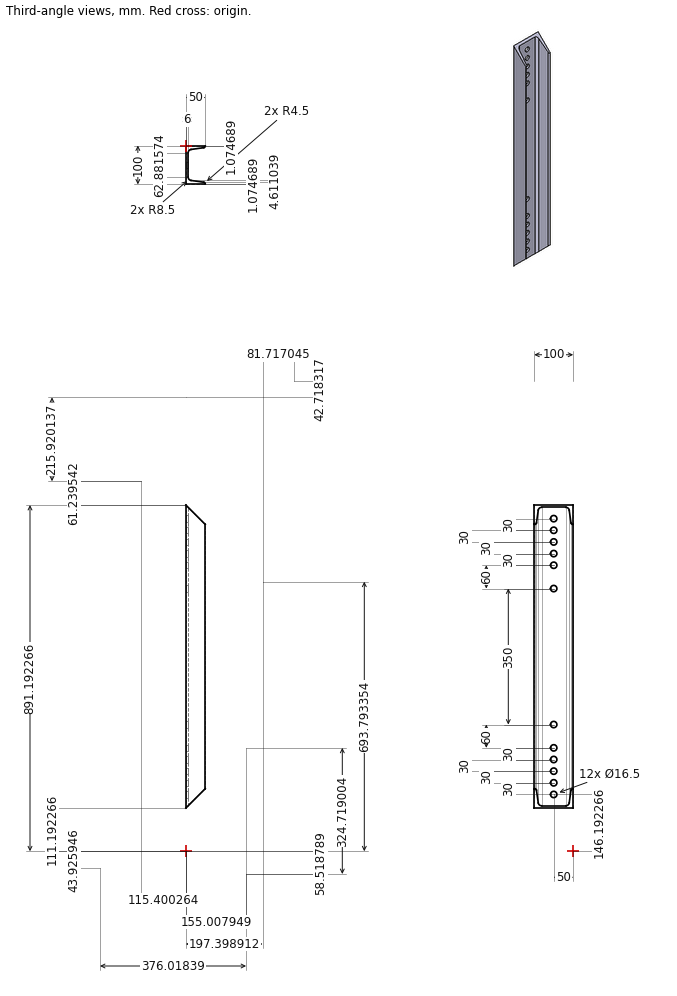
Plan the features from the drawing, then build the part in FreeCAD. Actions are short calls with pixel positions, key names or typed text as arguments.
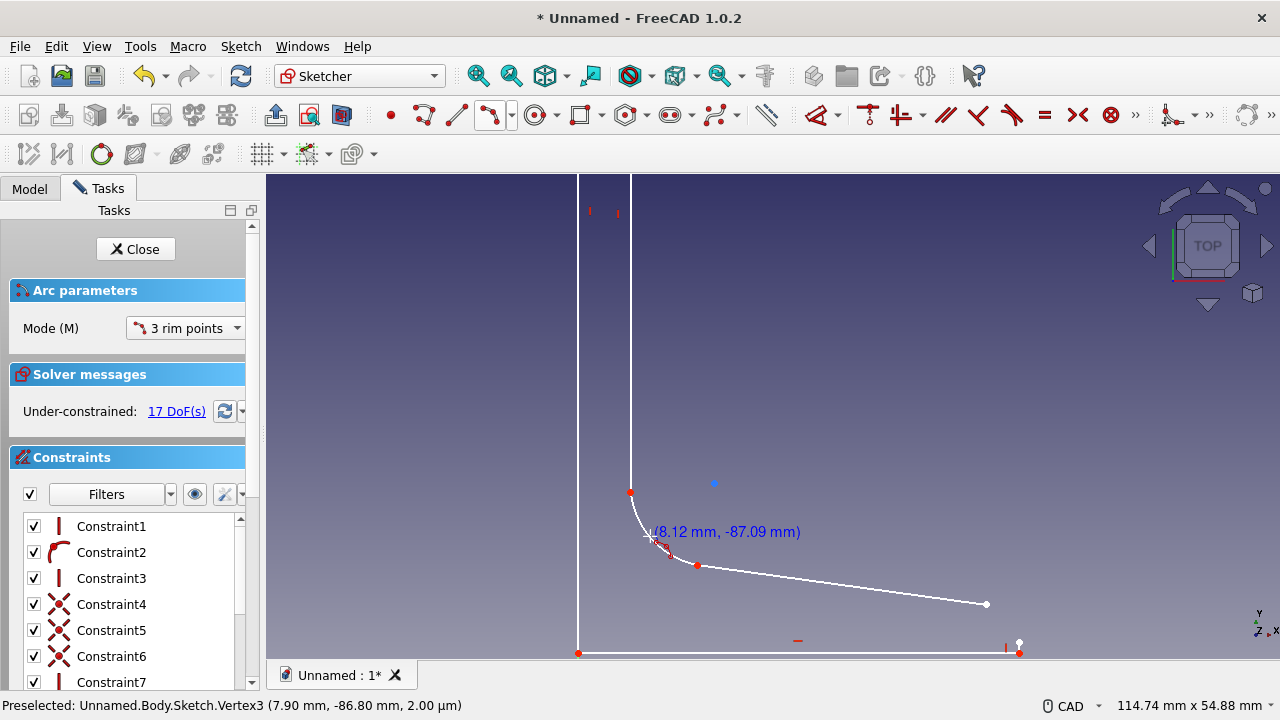
scroll(649, 537, down, 5)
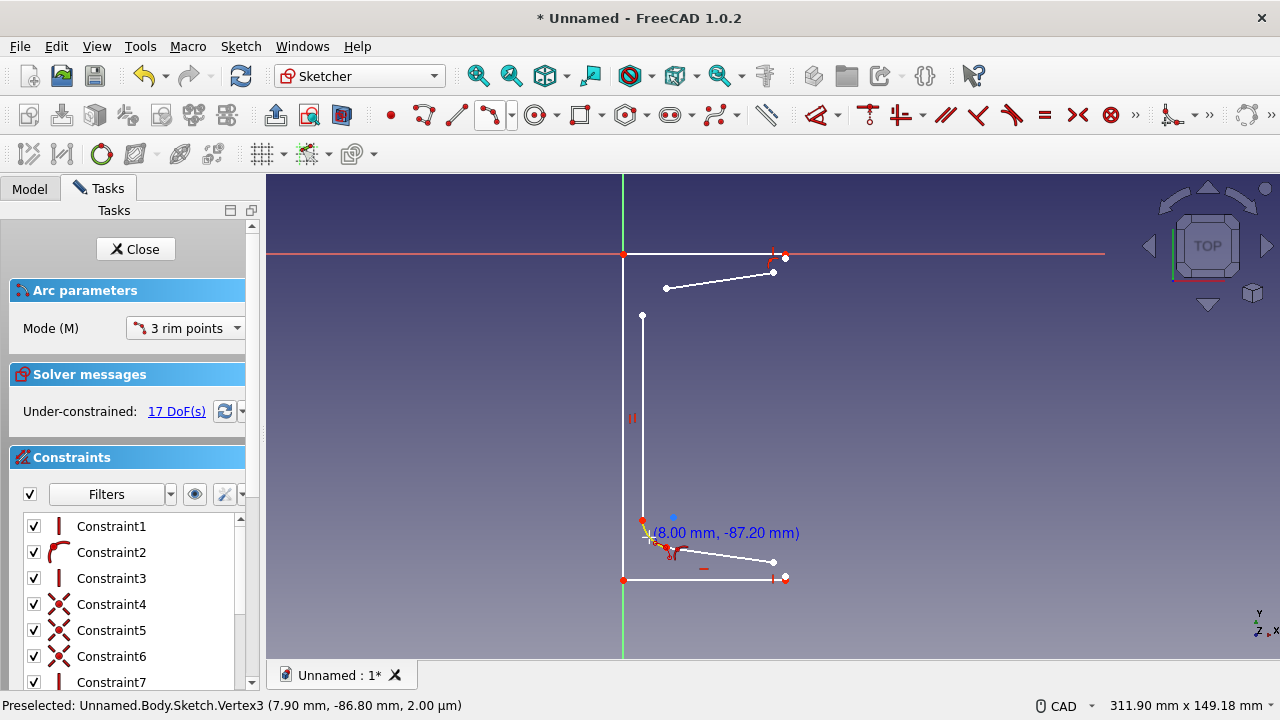
click(643, 316)
click(667, 289)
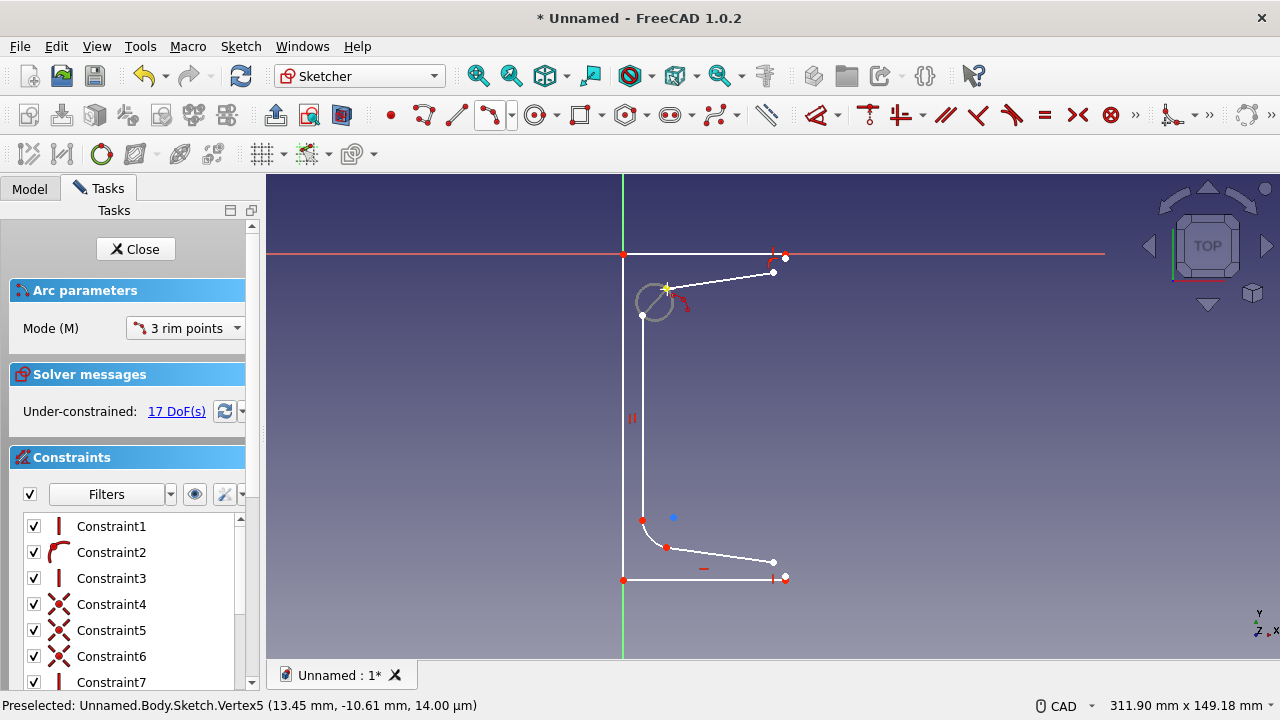
scroll(650, 297, up, 5)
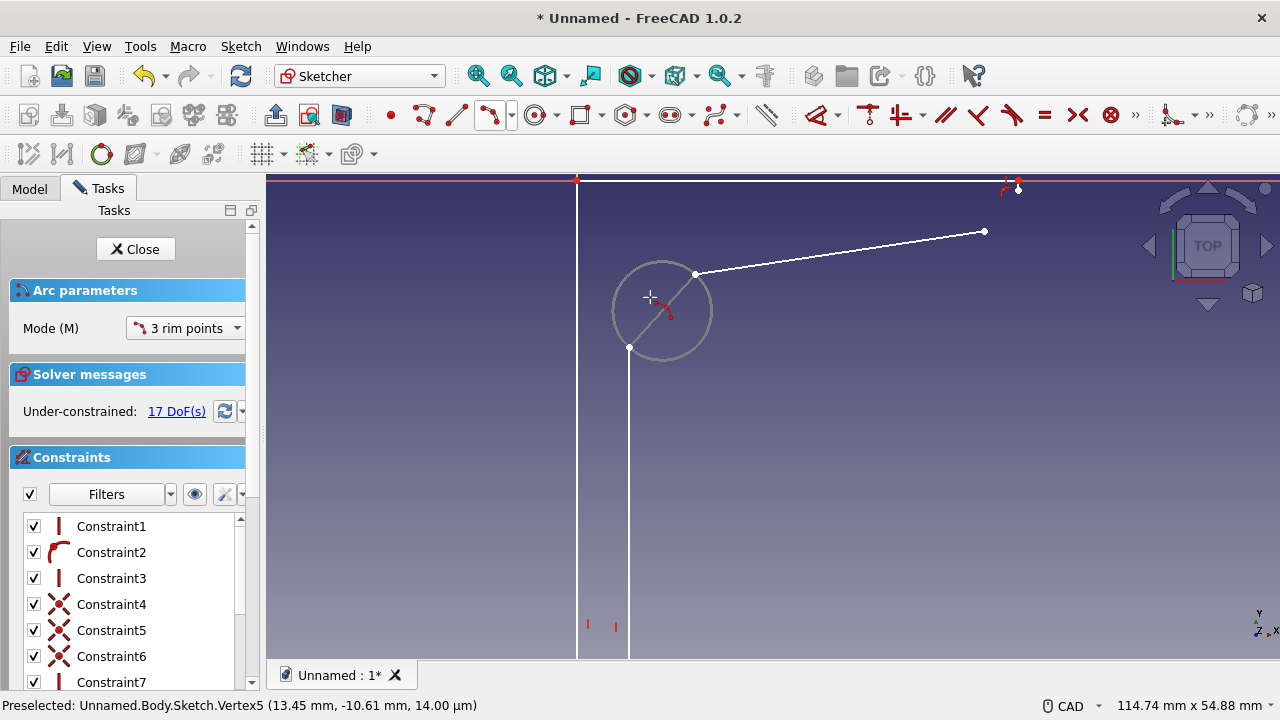
click(648, 295)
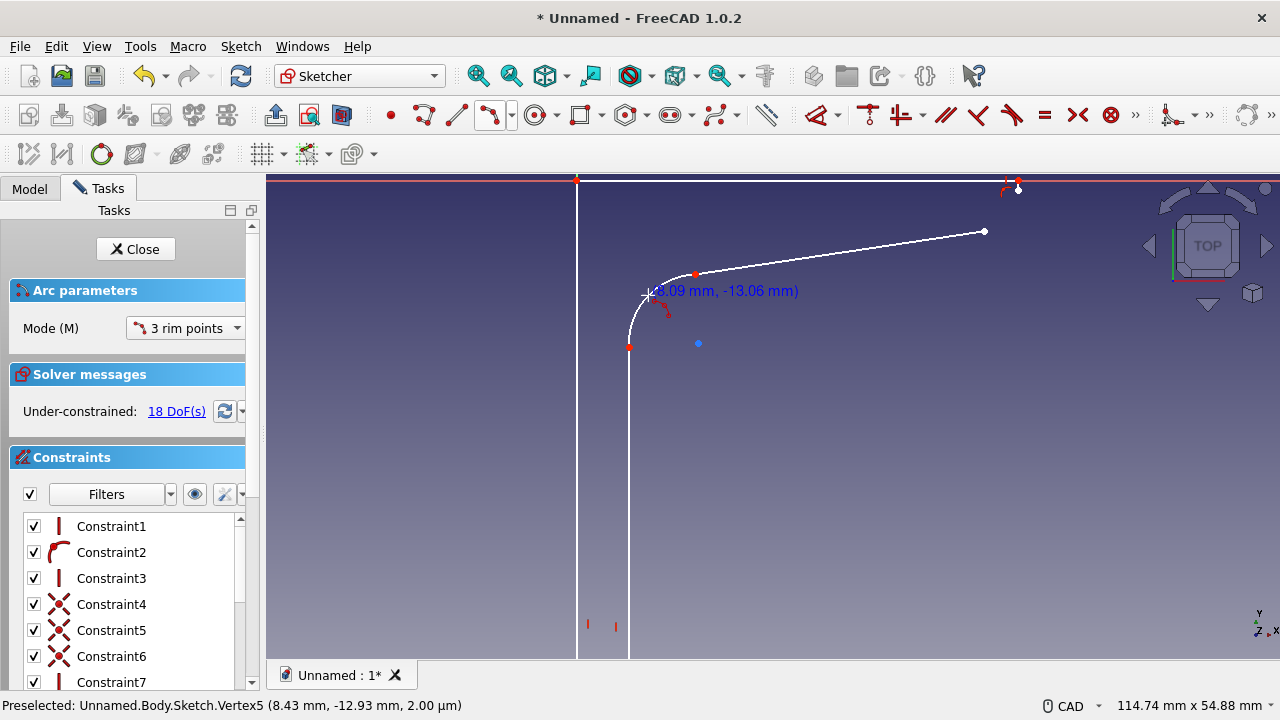
click(984, 231)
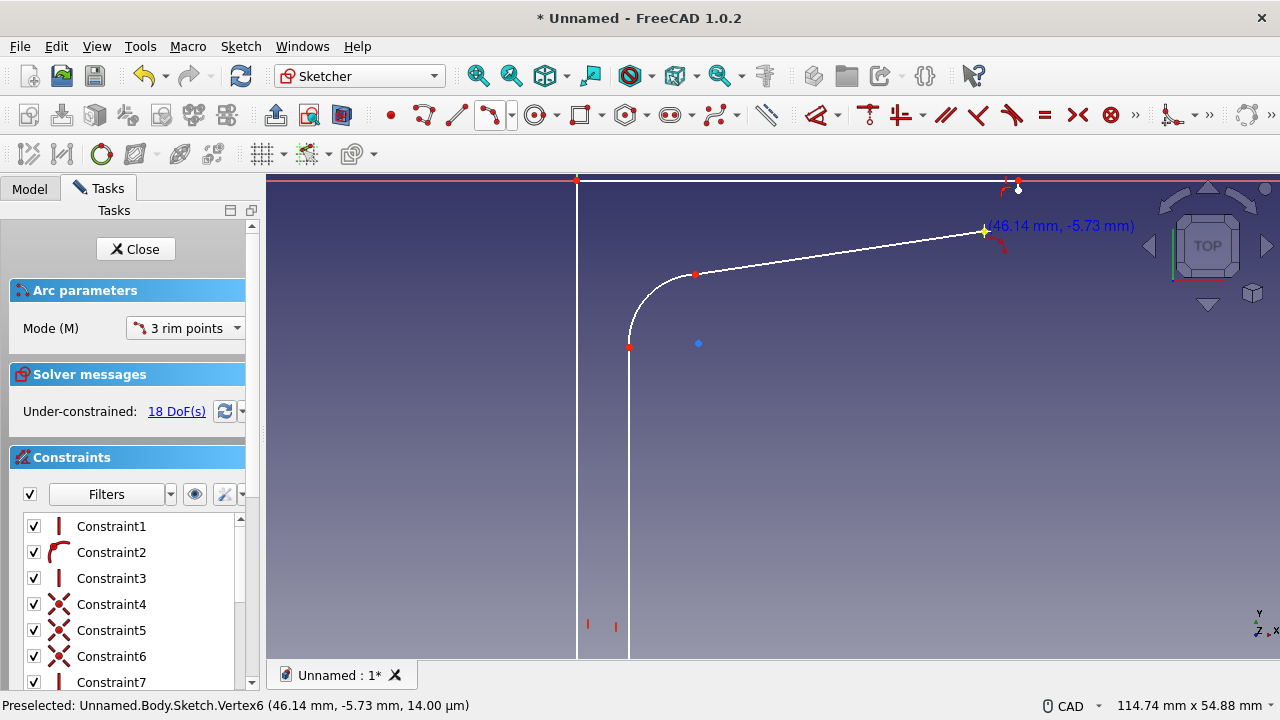
scroll(650, 297, down, 5)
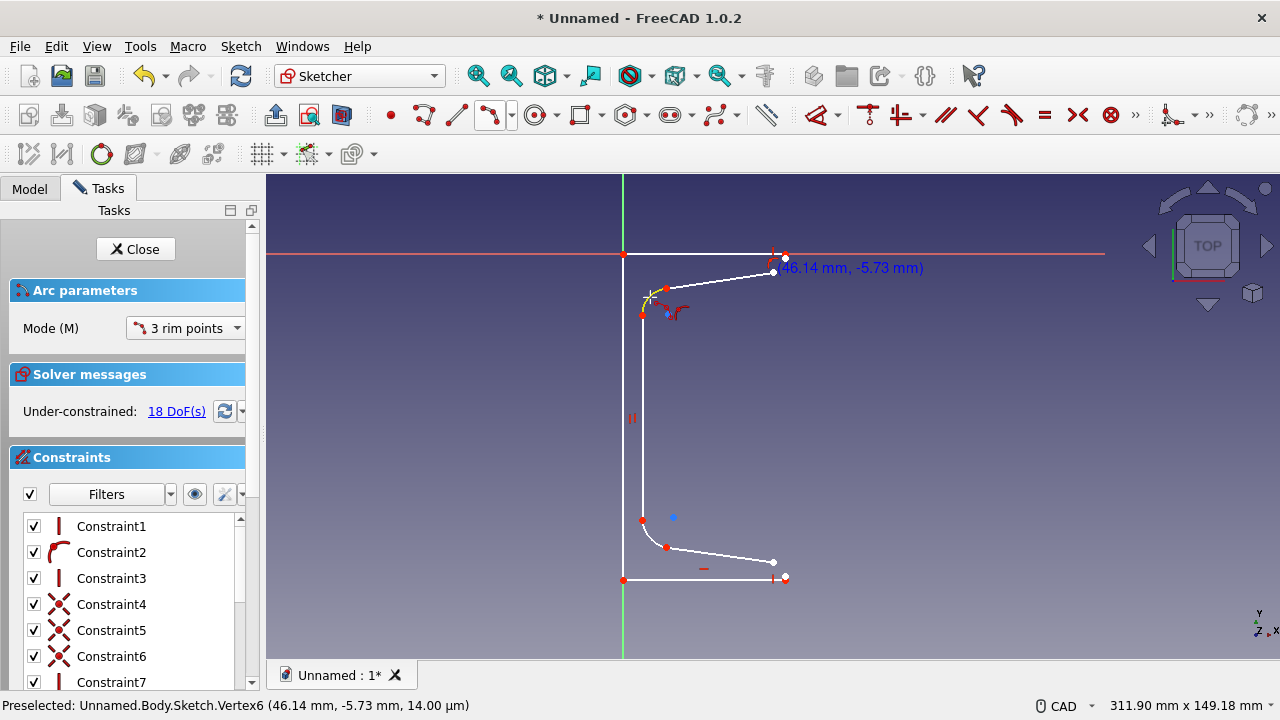
scroll(786, 258, up, 12)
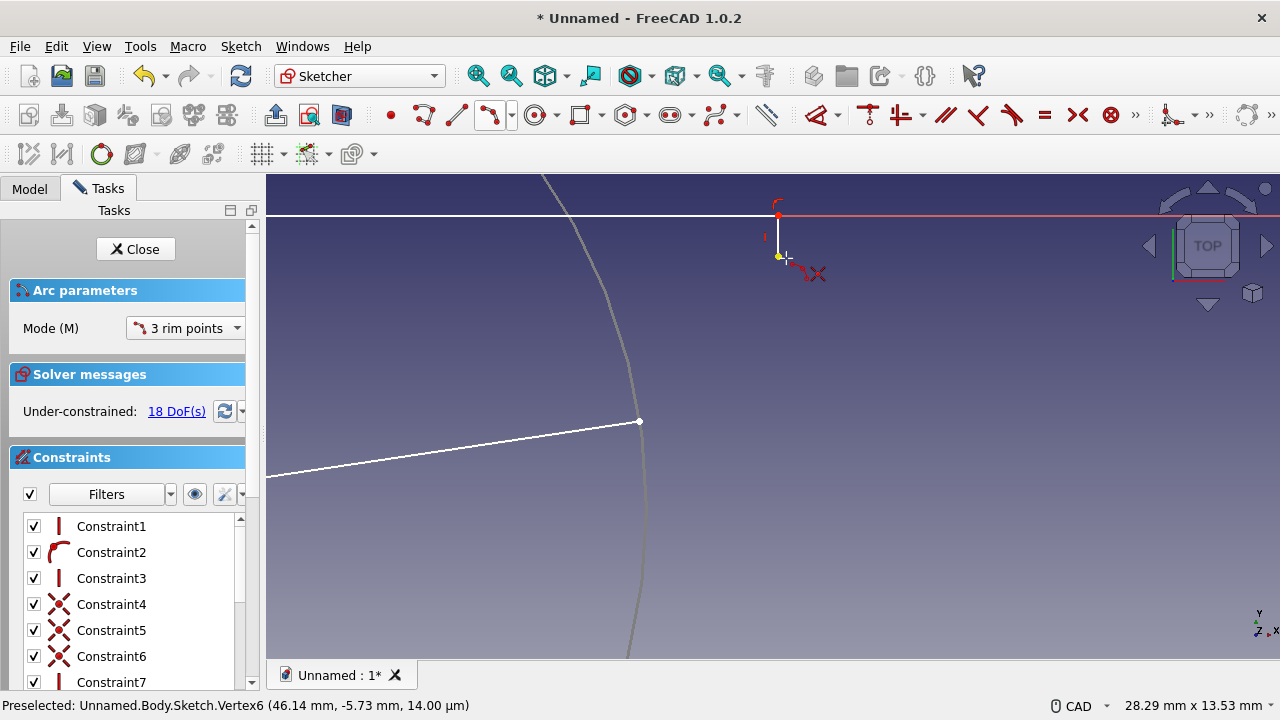
click(778, 257)
click(739, 360)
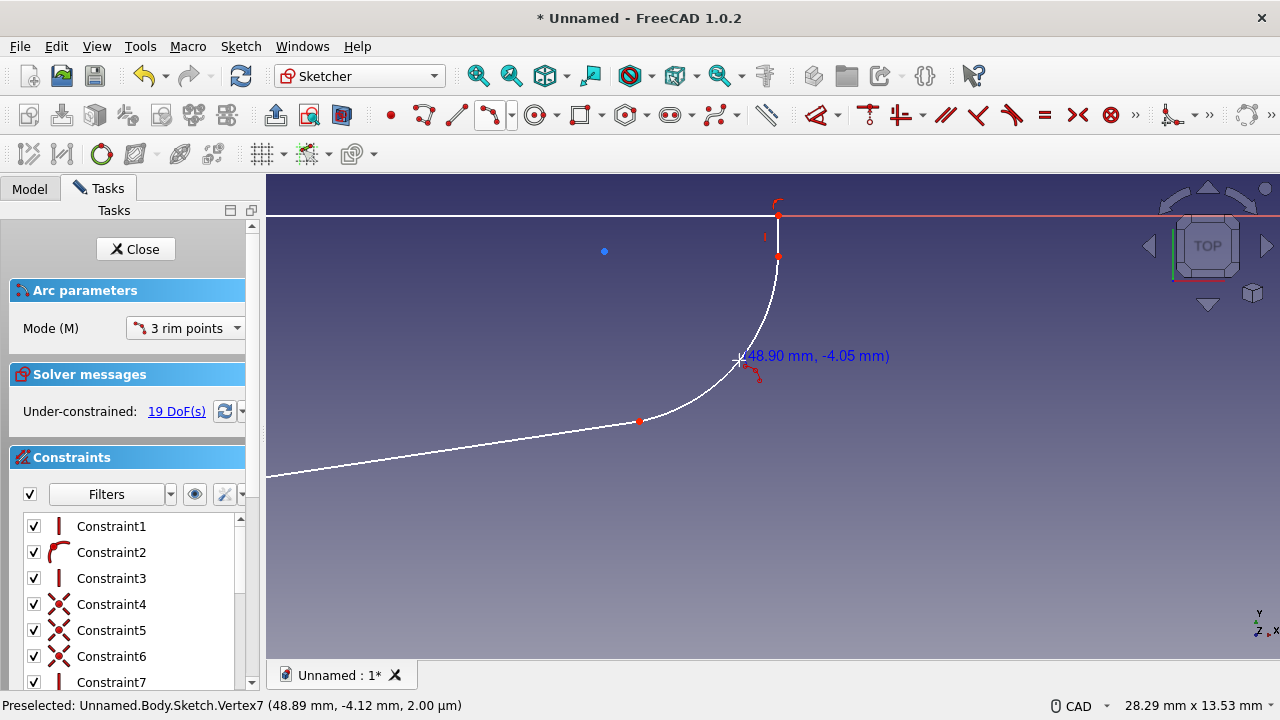
scroll(787, 258, down, 12)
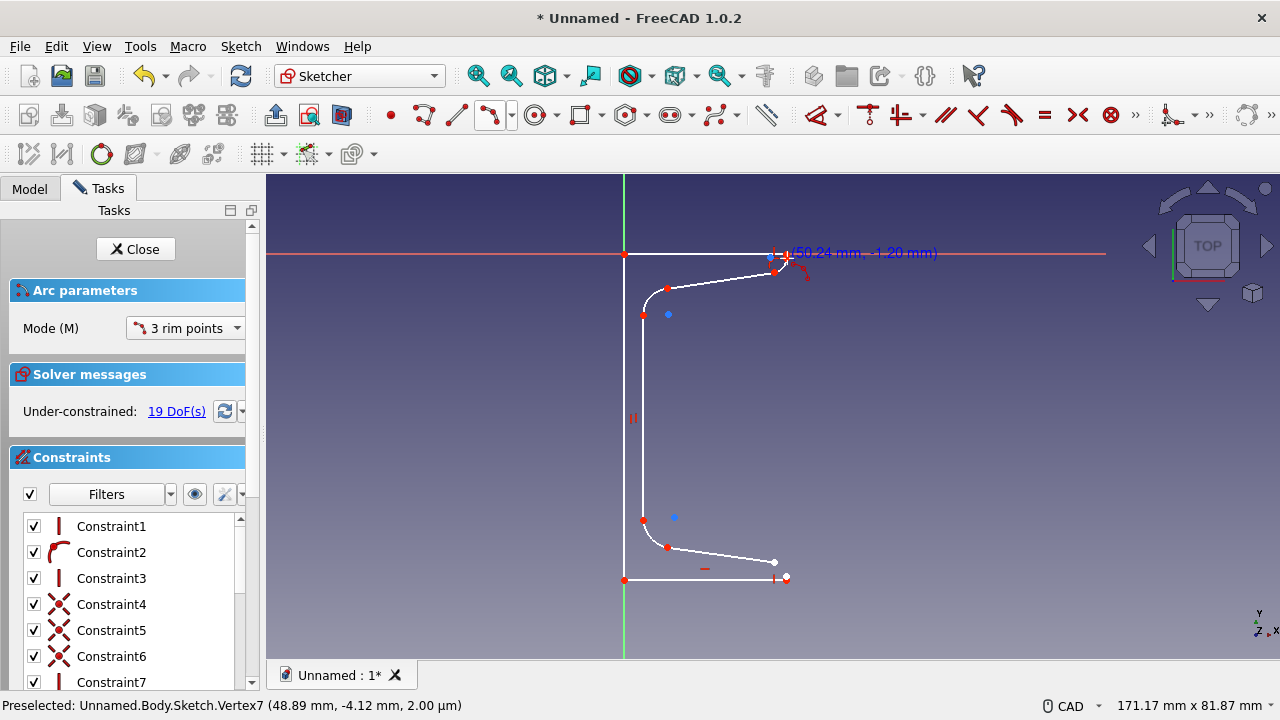
scroll(787, 576, up, 12)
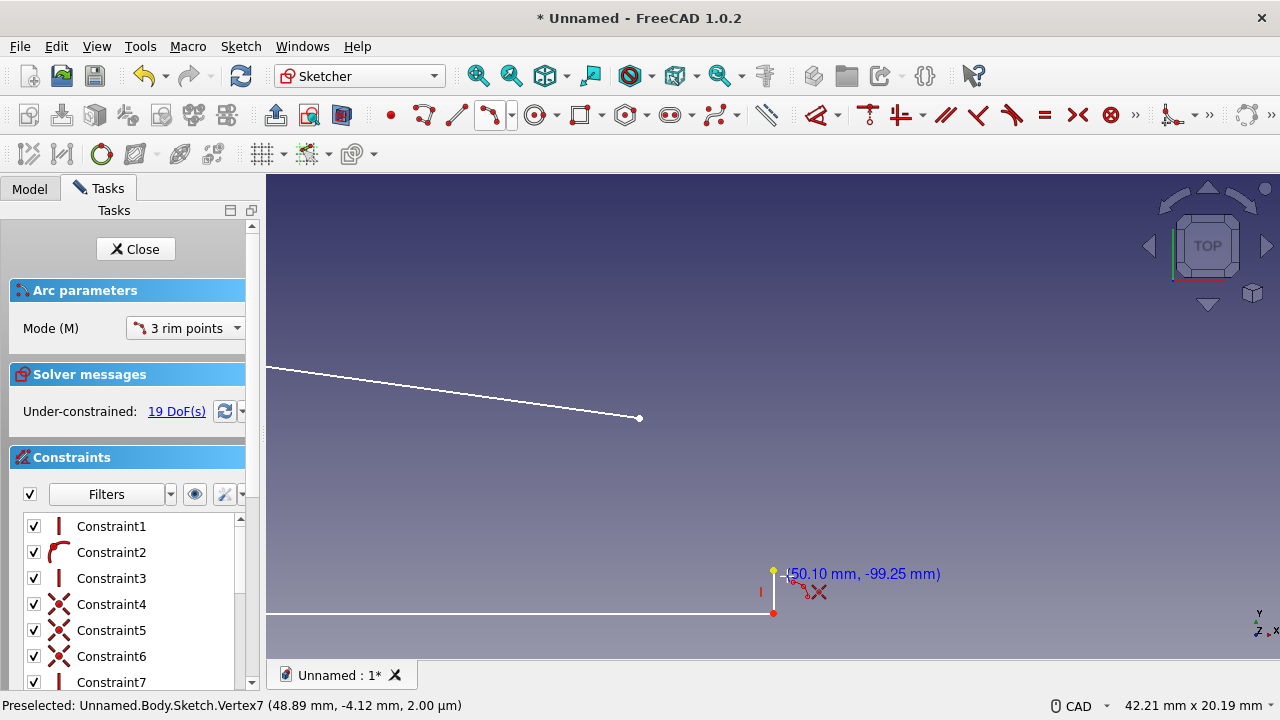
click(774, 570)